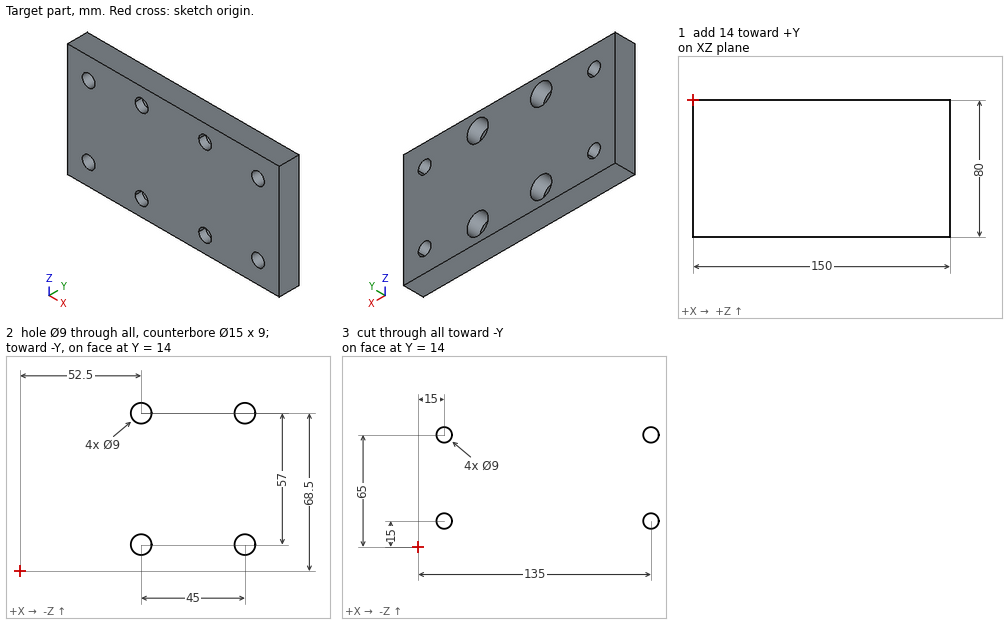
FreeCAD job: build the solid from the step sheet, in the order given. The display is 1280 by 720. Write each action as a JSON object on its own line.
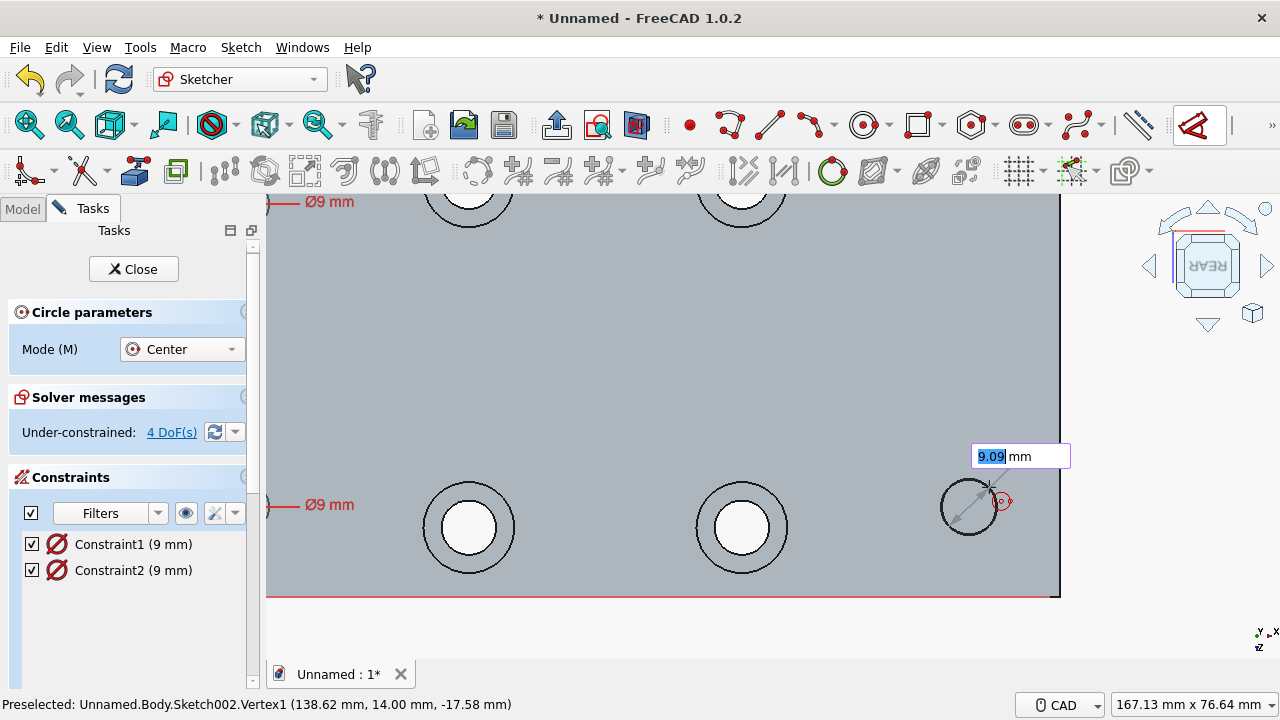
{"action": "type", "text": "9"}
{"action": "key", "text": "Return"}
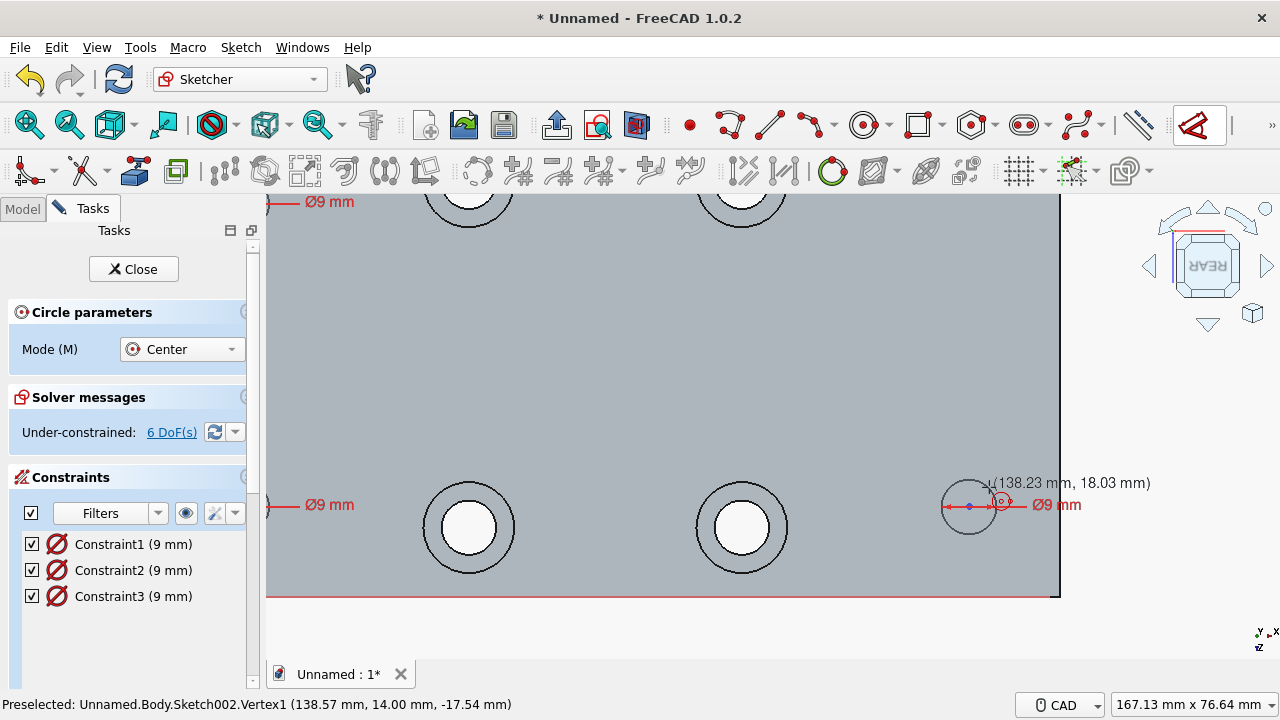
{"action": "scroll", "coordinate": [971, 508], "scroll_direction": "down", "scroll_amount": 2}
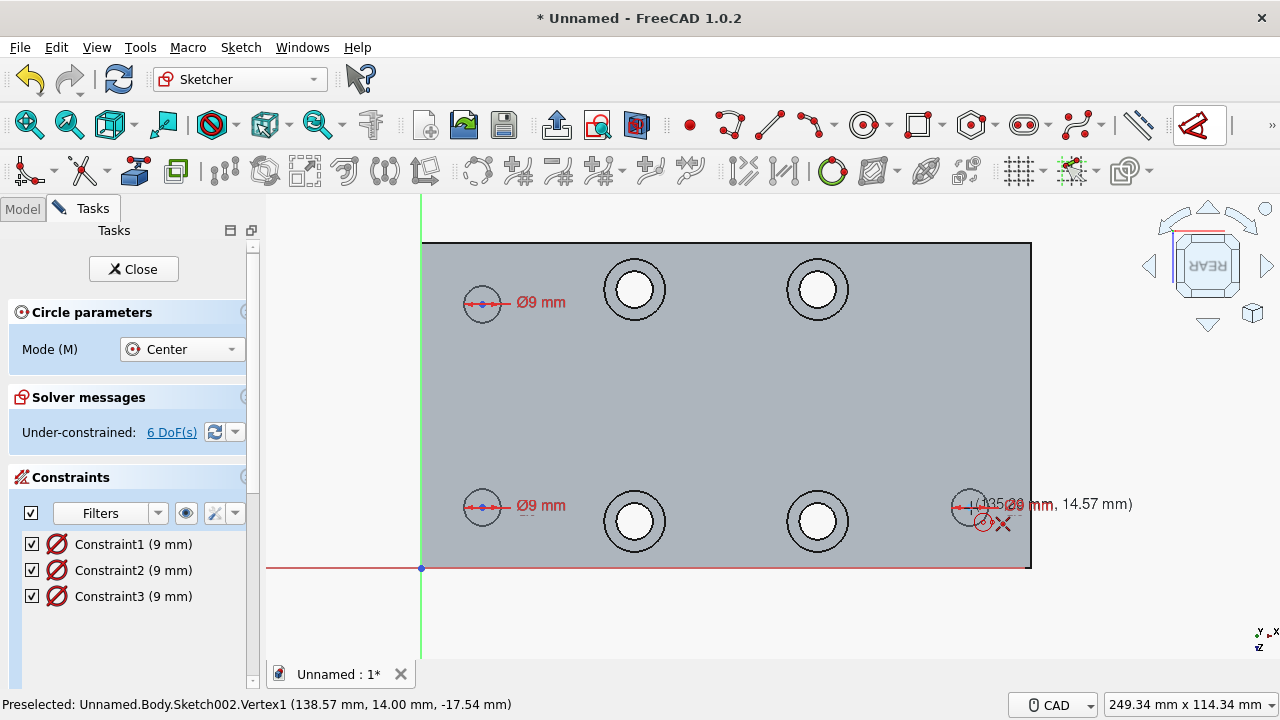
{"action": "scroll", "coordinate": [970, 304], "scroll_direction": "up", "scroll_amount": 2}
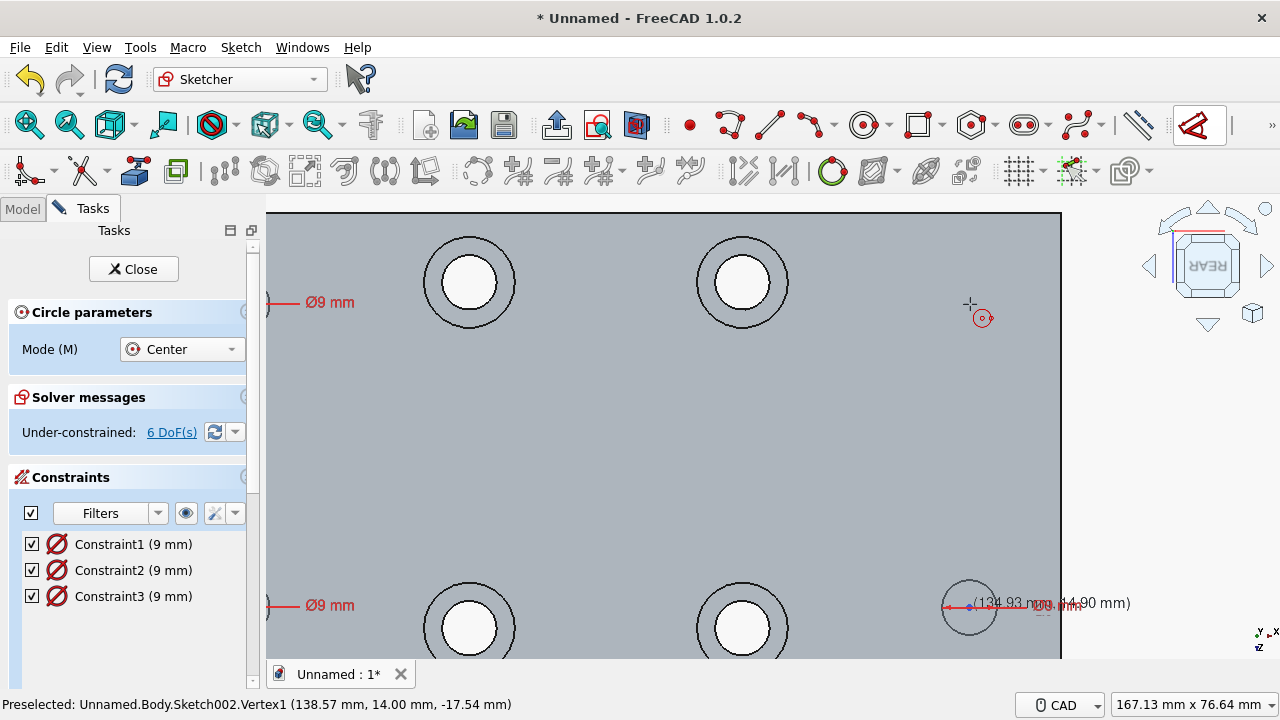
{"action": "left_click", "coordinate": [970, 304]}
{"action": "mouse_move", "coordinate": [989, 284]}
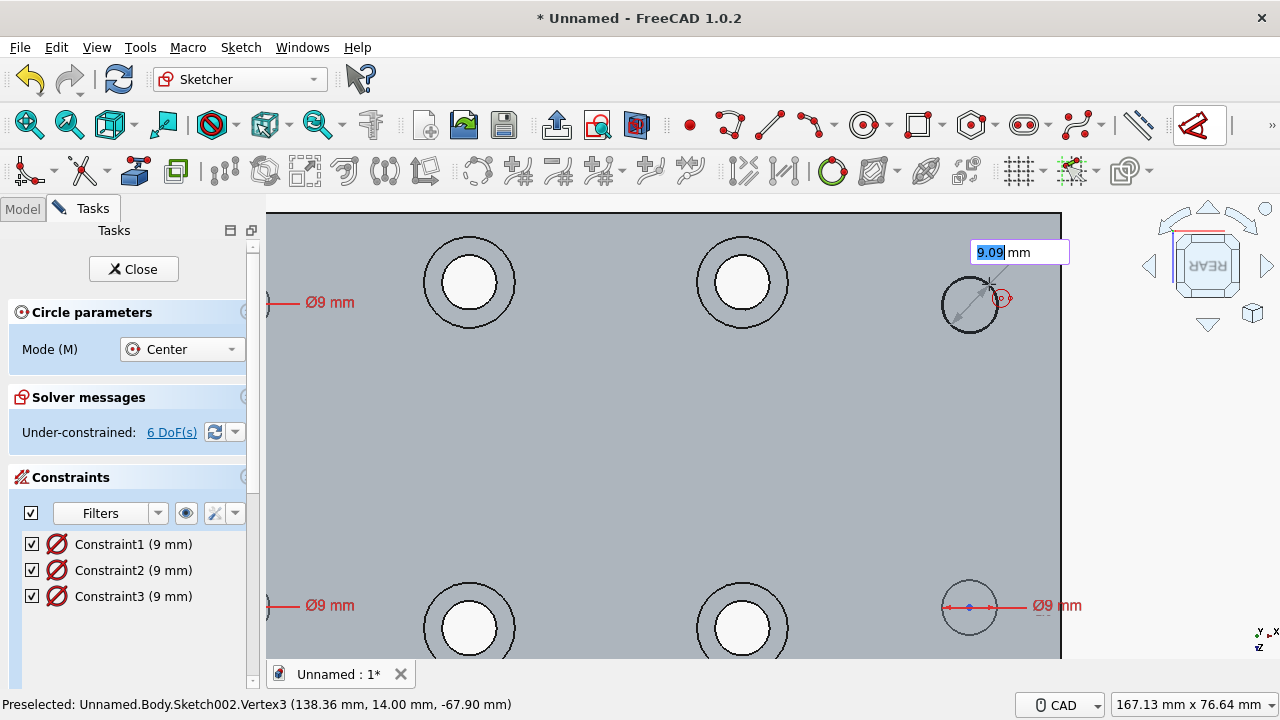
{"action": "type", "text": "9"}
{"action": "key", "text": "Return"}
{"action": "key", "text": "Escape"}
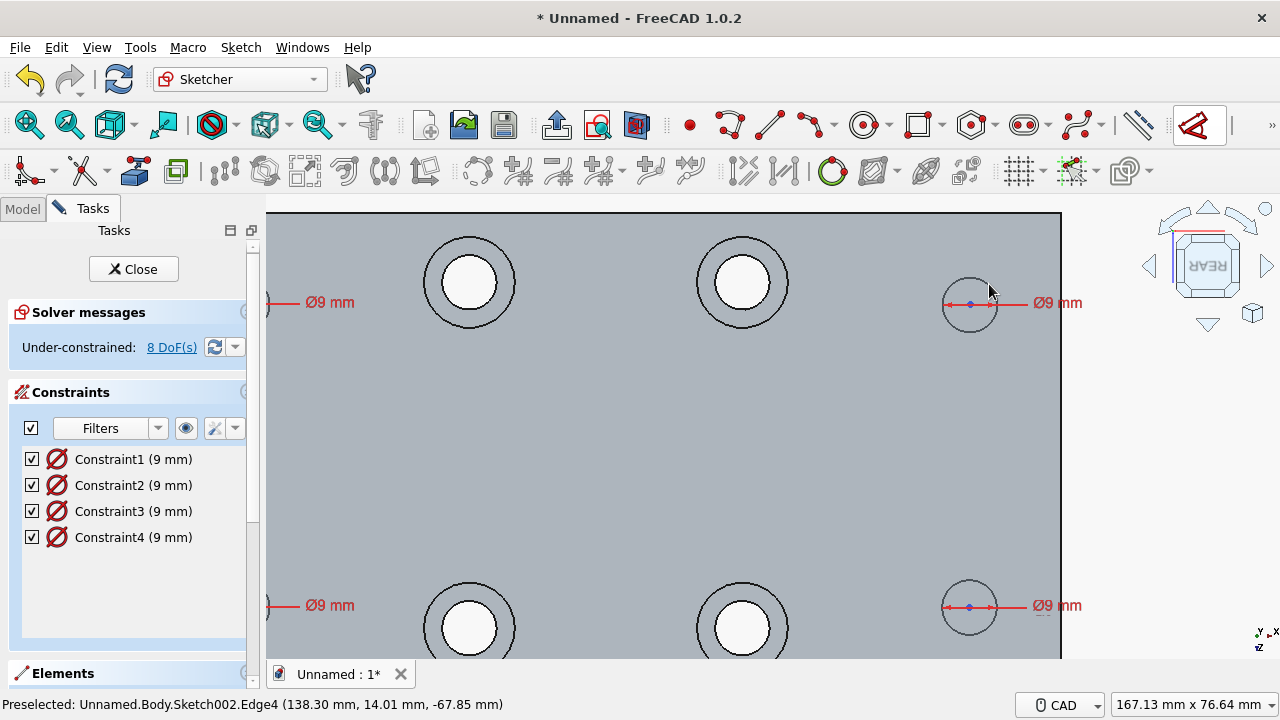
{"action": "scroll", "coordinate": [970, 303], "scroll_direction": "down", "scroll_amount": 2}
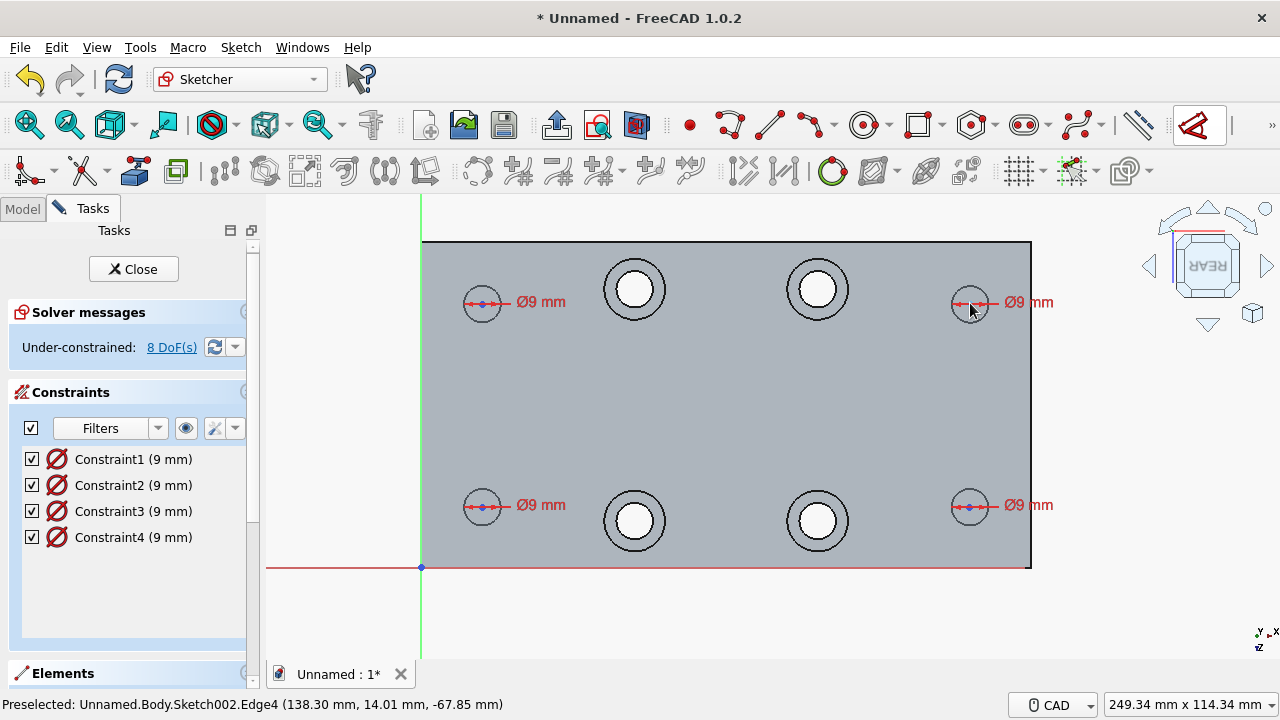
{"action": "left_click", "coordinate": [482, 304]}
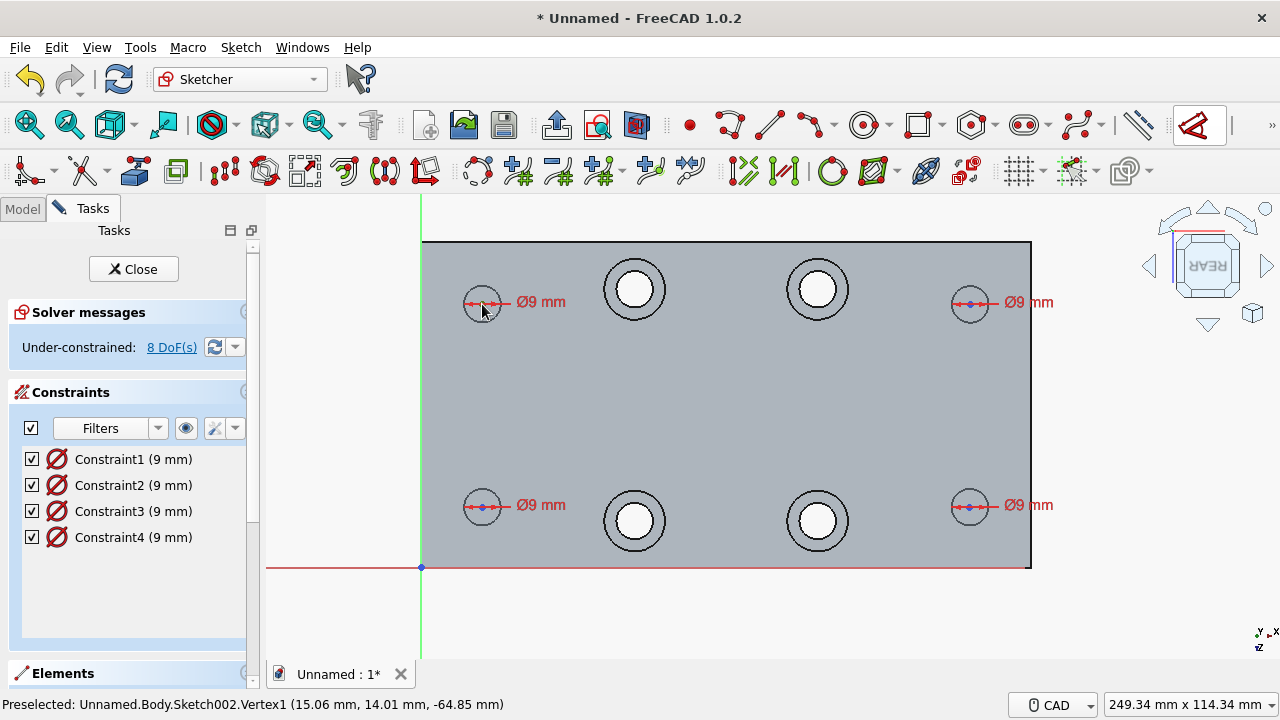
{"action": "left_click", "coordinate": [482, 507]}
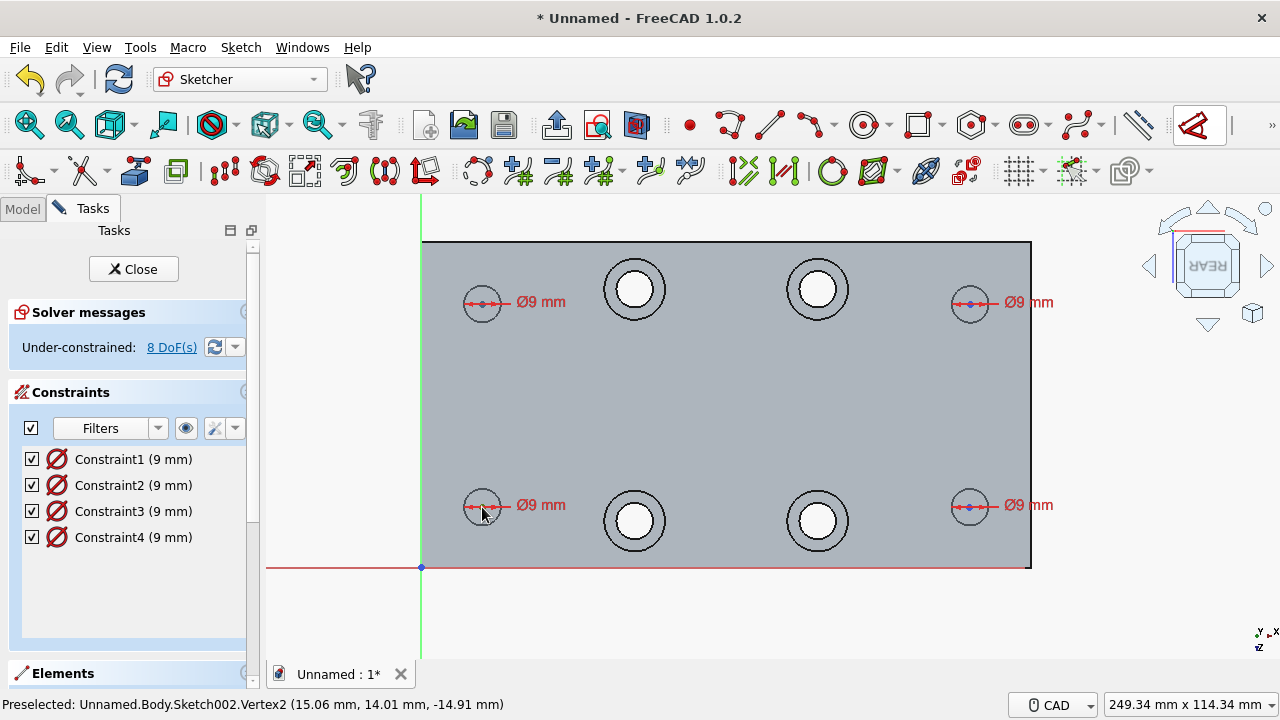
{"action": "key", "text": "v"}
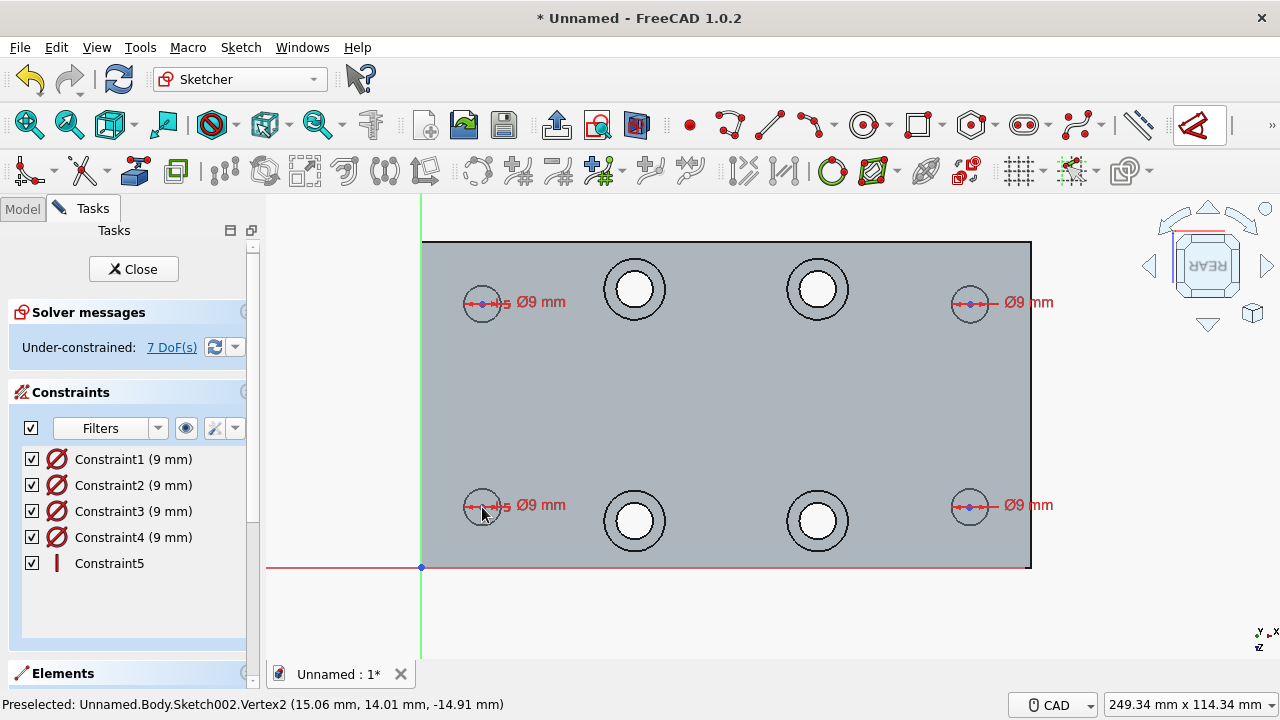
{"action": "left_click", "coordinate": [482, 507]}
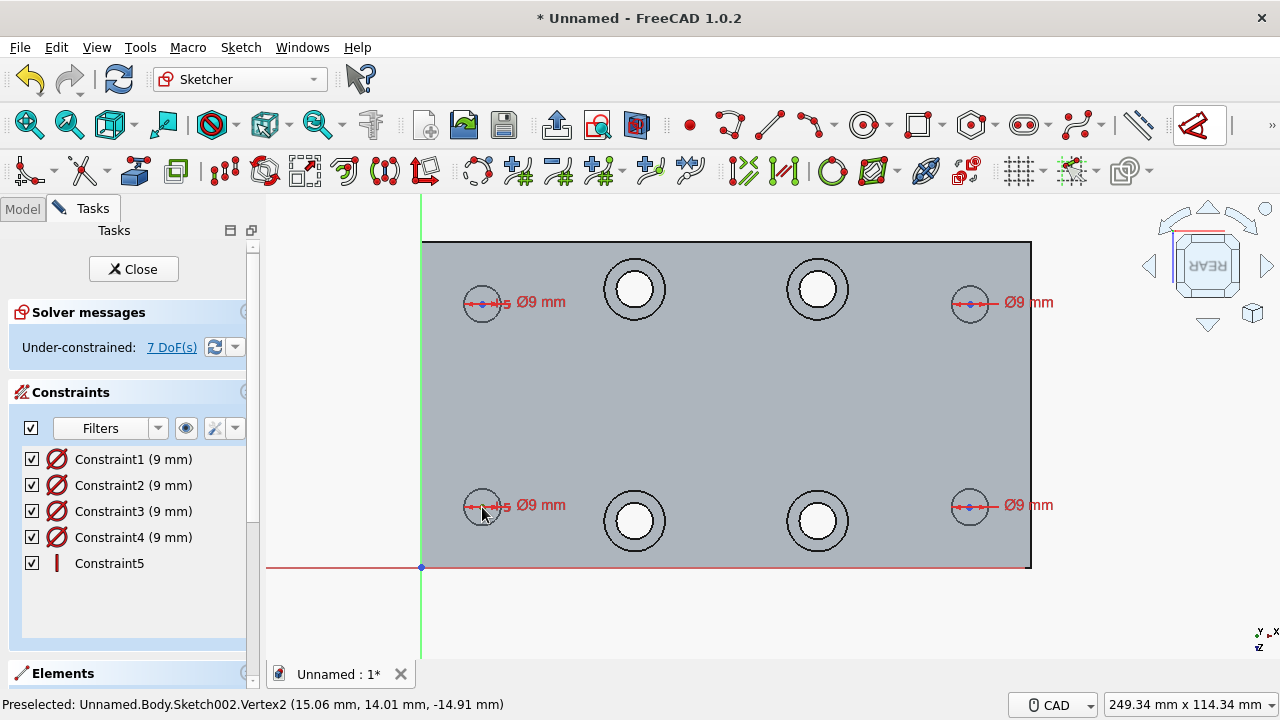
{"action": "left_click", "coordinate": [970, 507]}